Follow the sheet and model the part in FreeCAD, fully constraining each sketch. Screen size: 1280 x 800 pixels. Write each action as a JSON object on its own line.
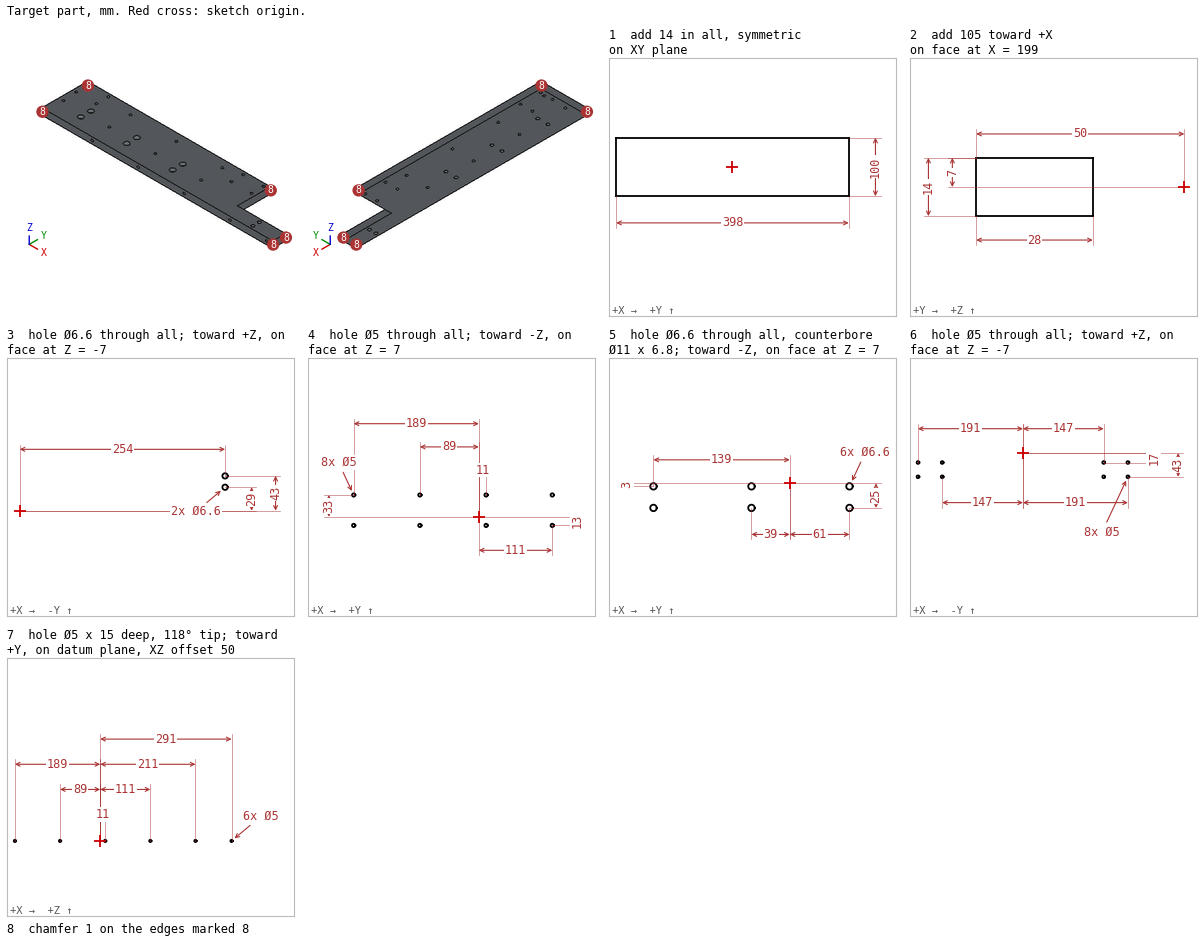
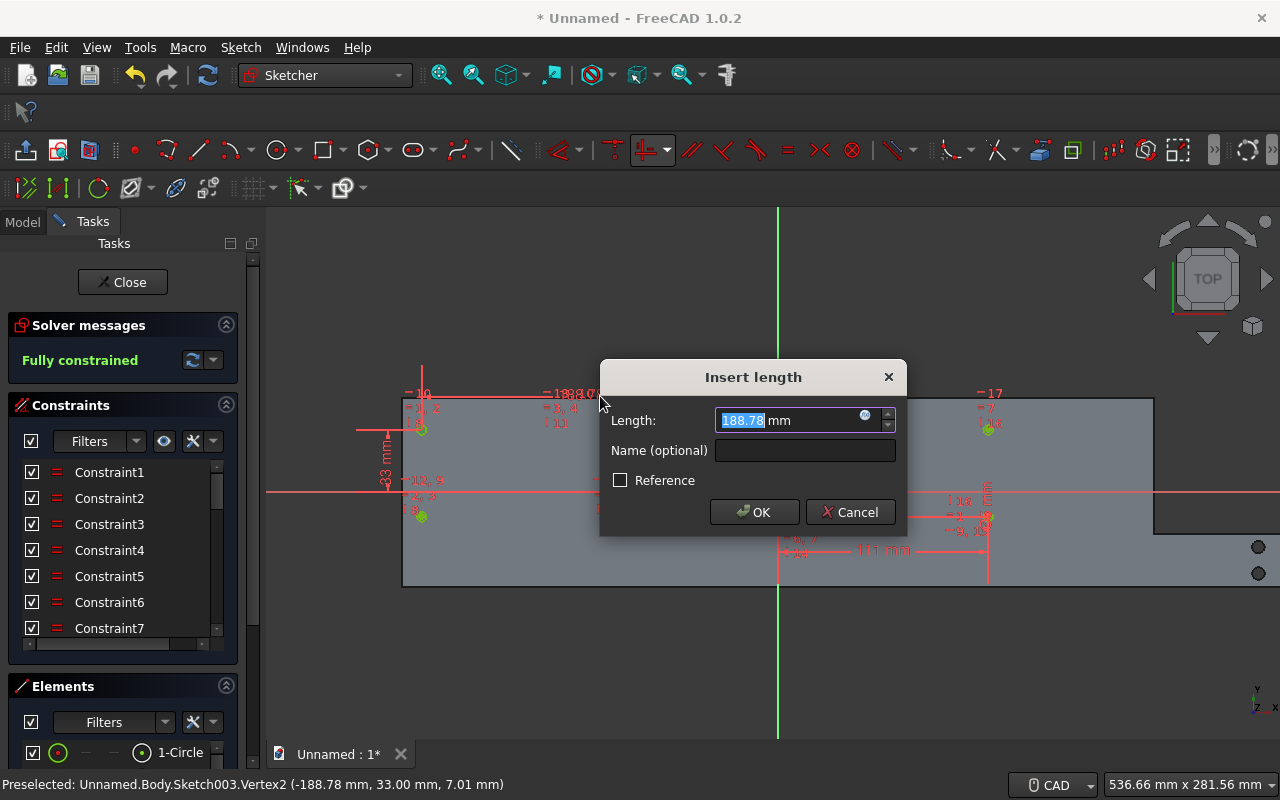
{"action": "type", "text": "189"}
{"action": "key", "text": "Return"}
{"action": "key", "text": "Escape"}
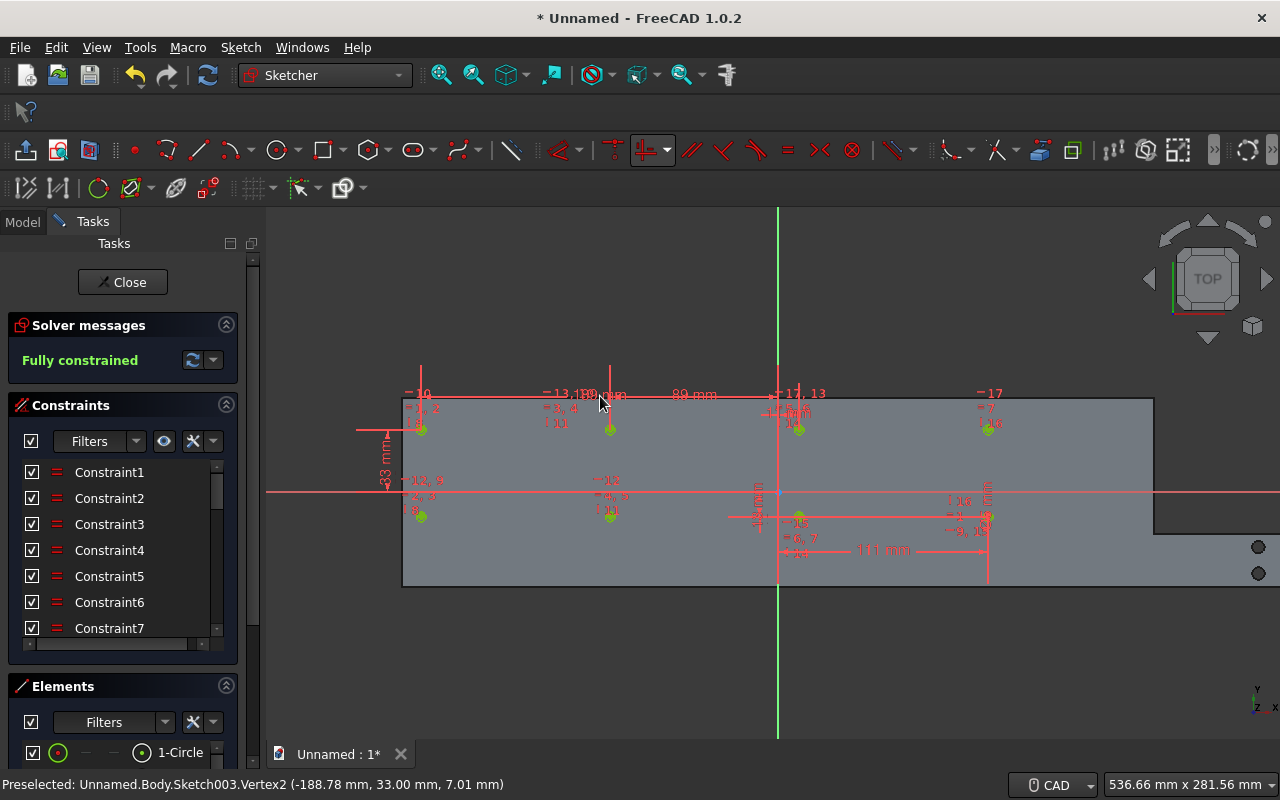
{"action": "left_click", "coordinate": [123, 282]}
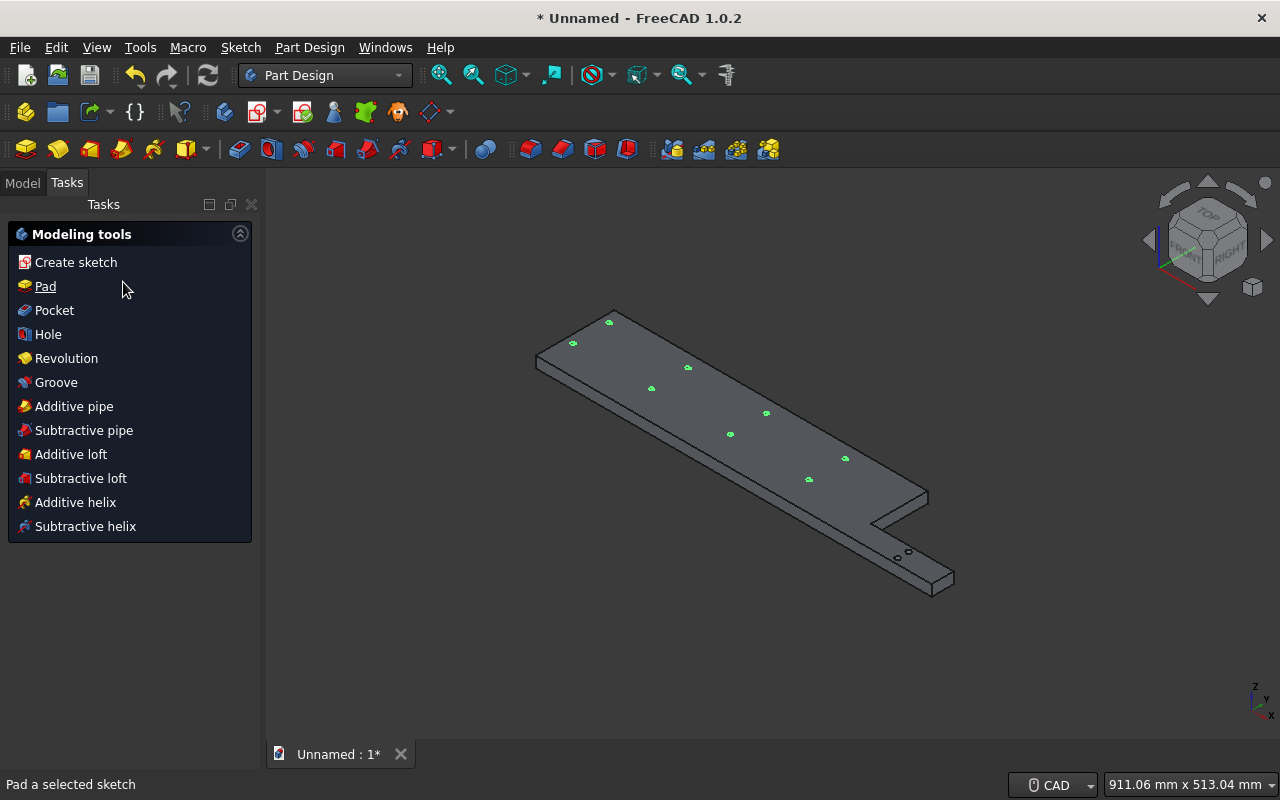
{"action": "left_click", "coordinate": [272, 150]}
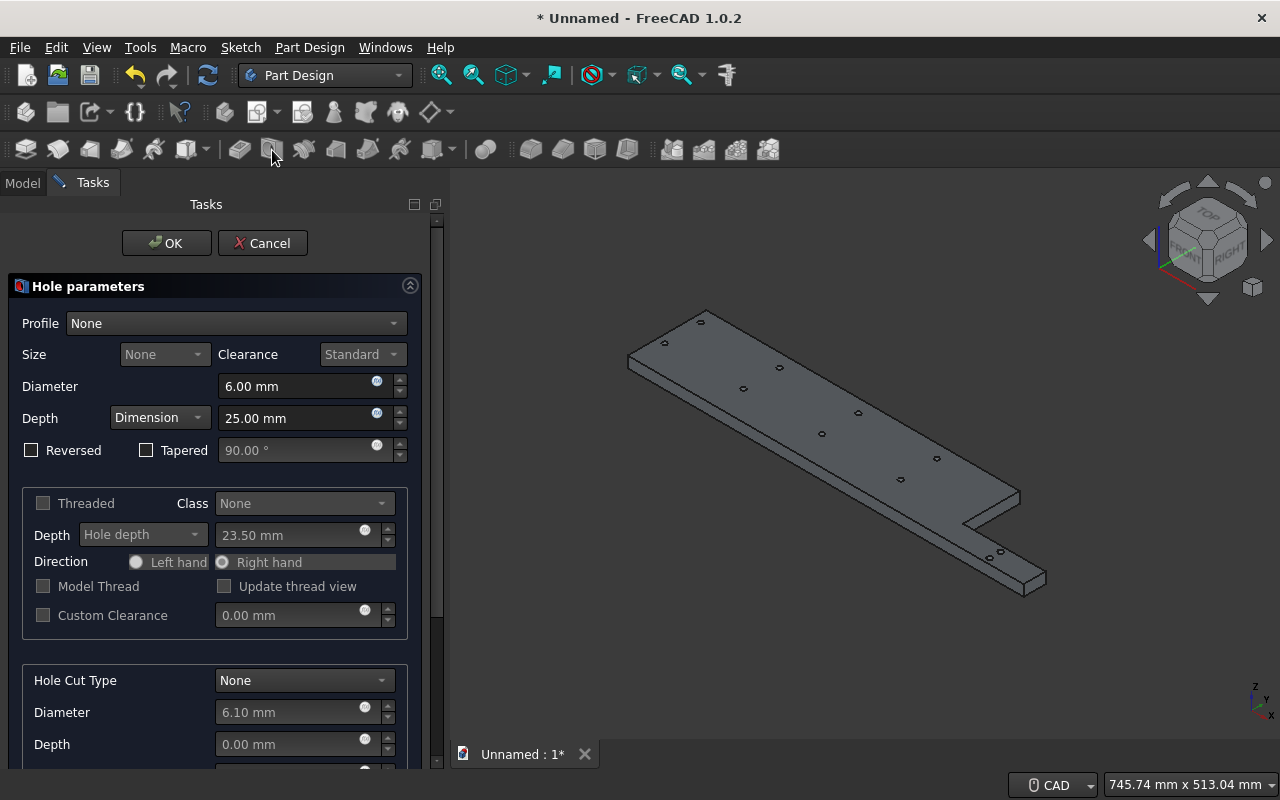
{"action": "triple_click", "coordinate": [305, 386]}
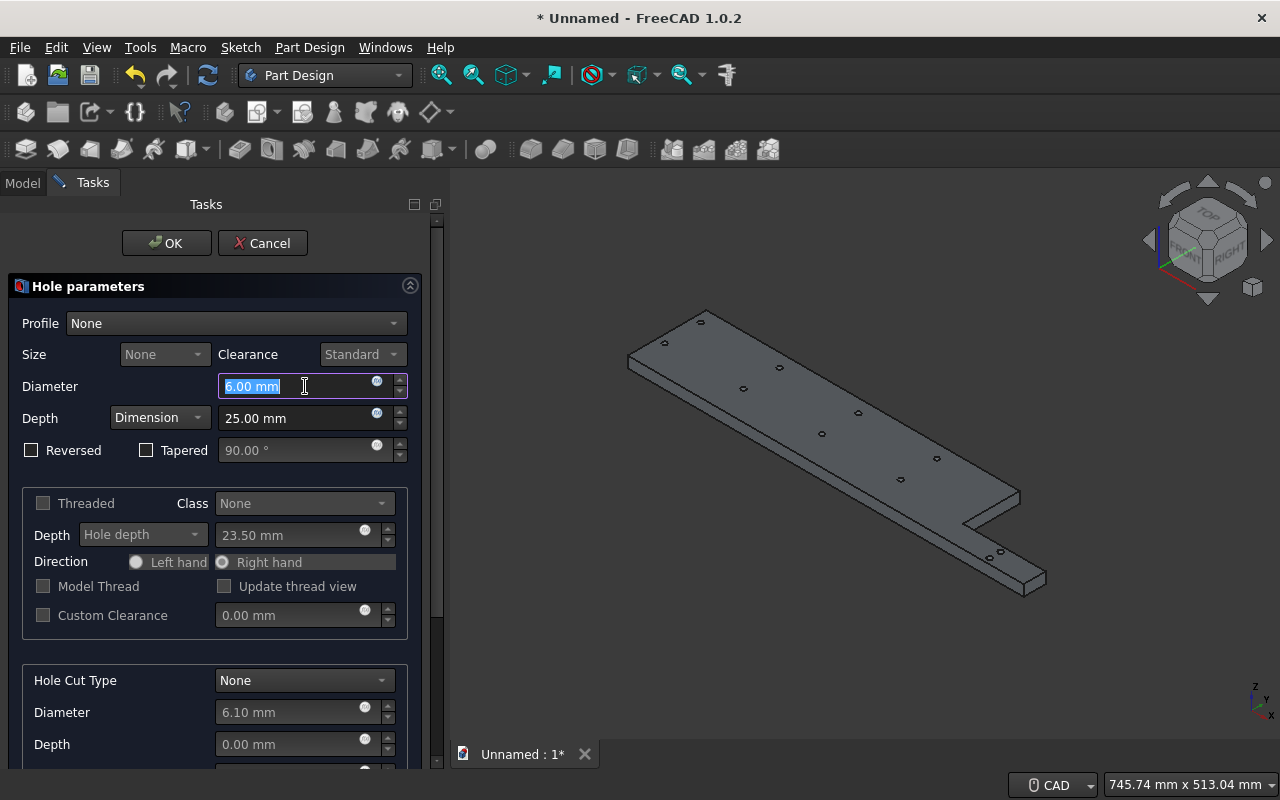
{"action": "type", "text": "5"}
{"action": "key", "text": "Tab"}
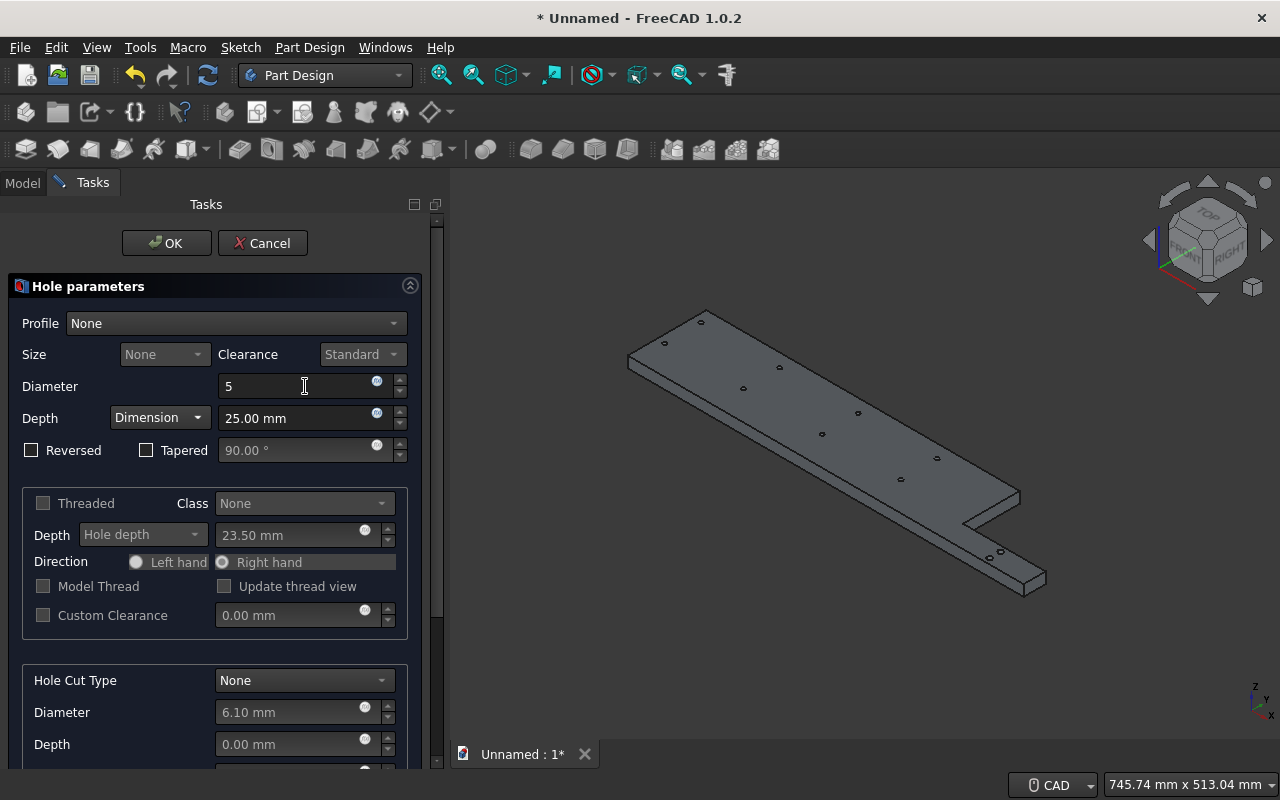
{"action": "left_click", "coordinate": [161, 418]}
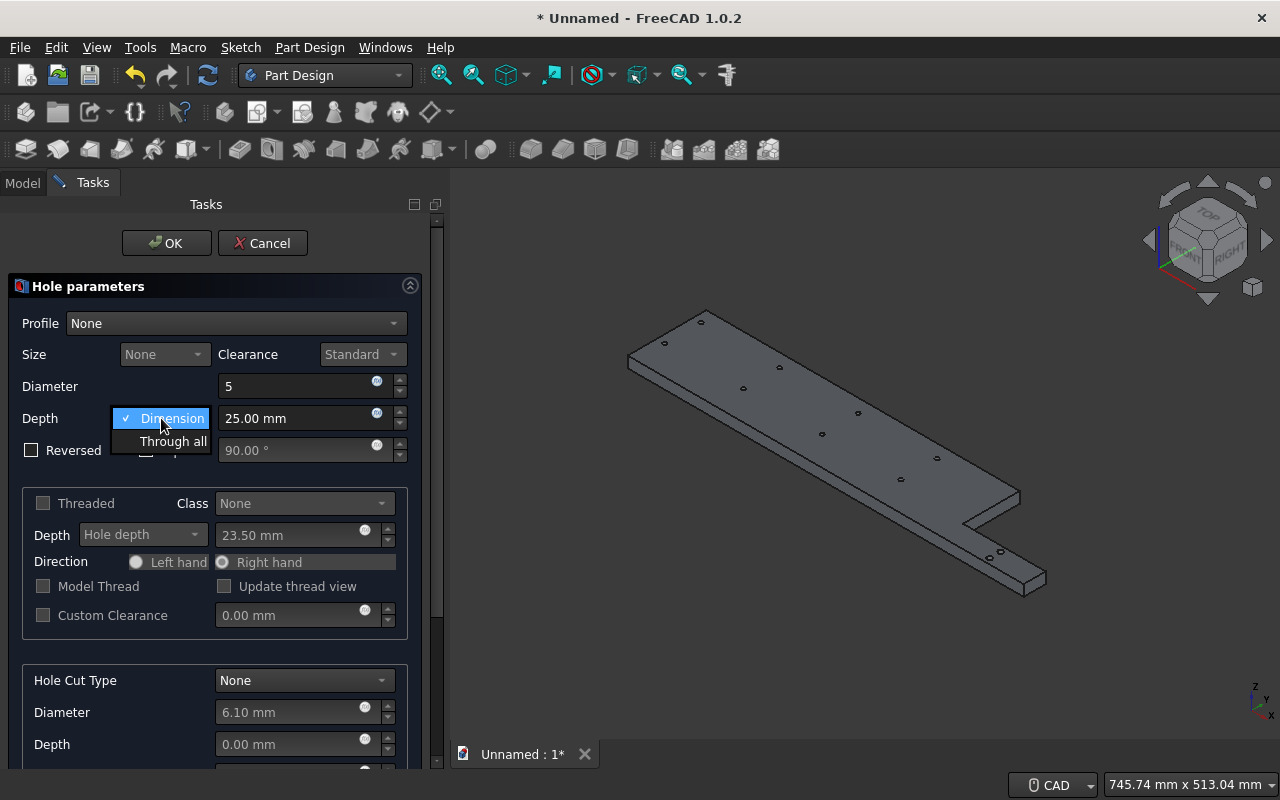
{"action": "left_click", "coordinate": [160, 442]}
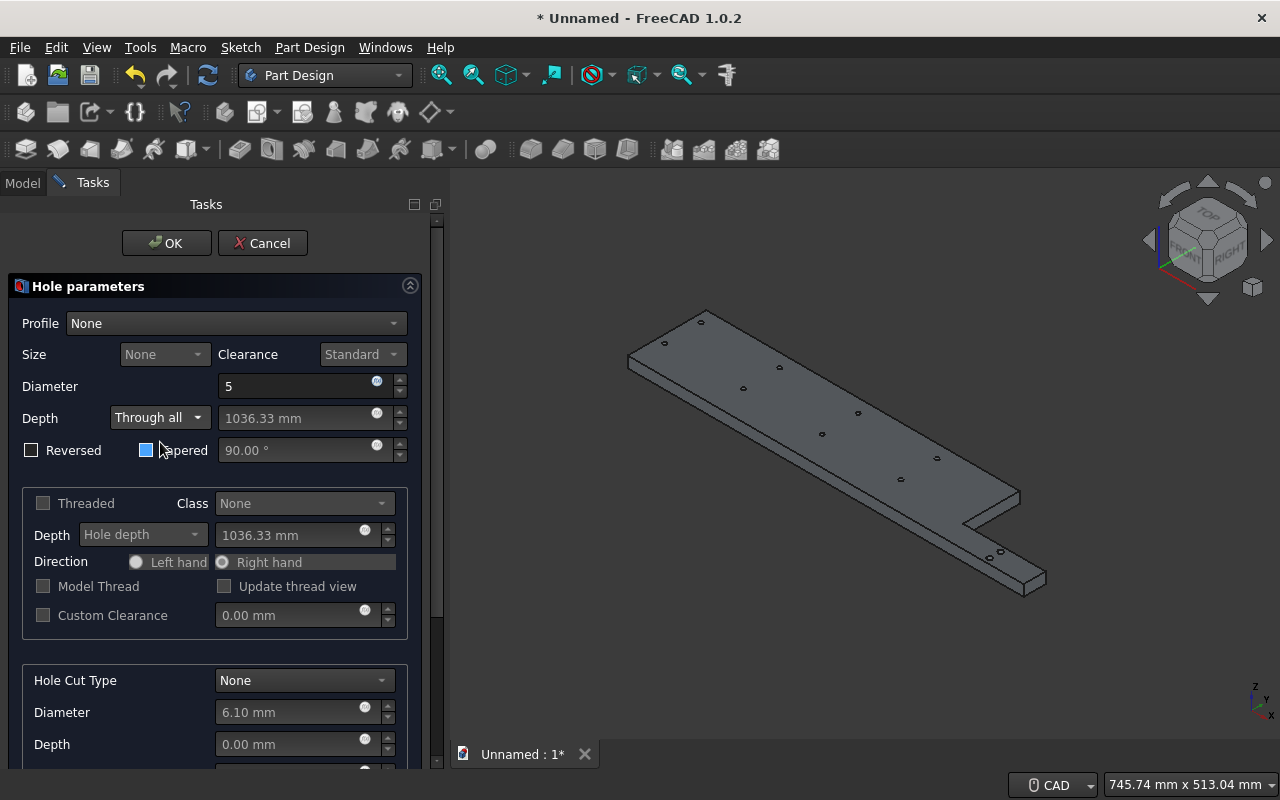
{"action": "left_click", "coordinate": [167, 243]}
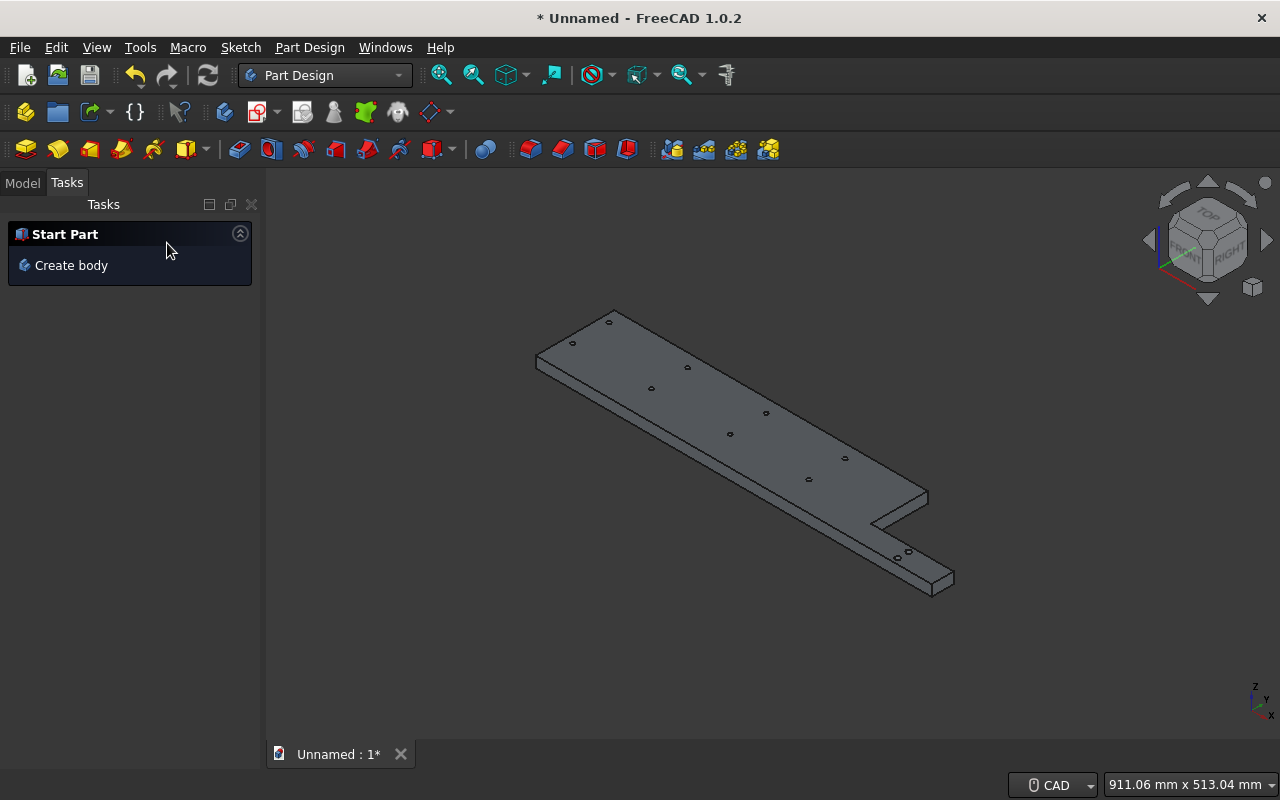
{"action": "left_click", "coordinate": [773, 446]}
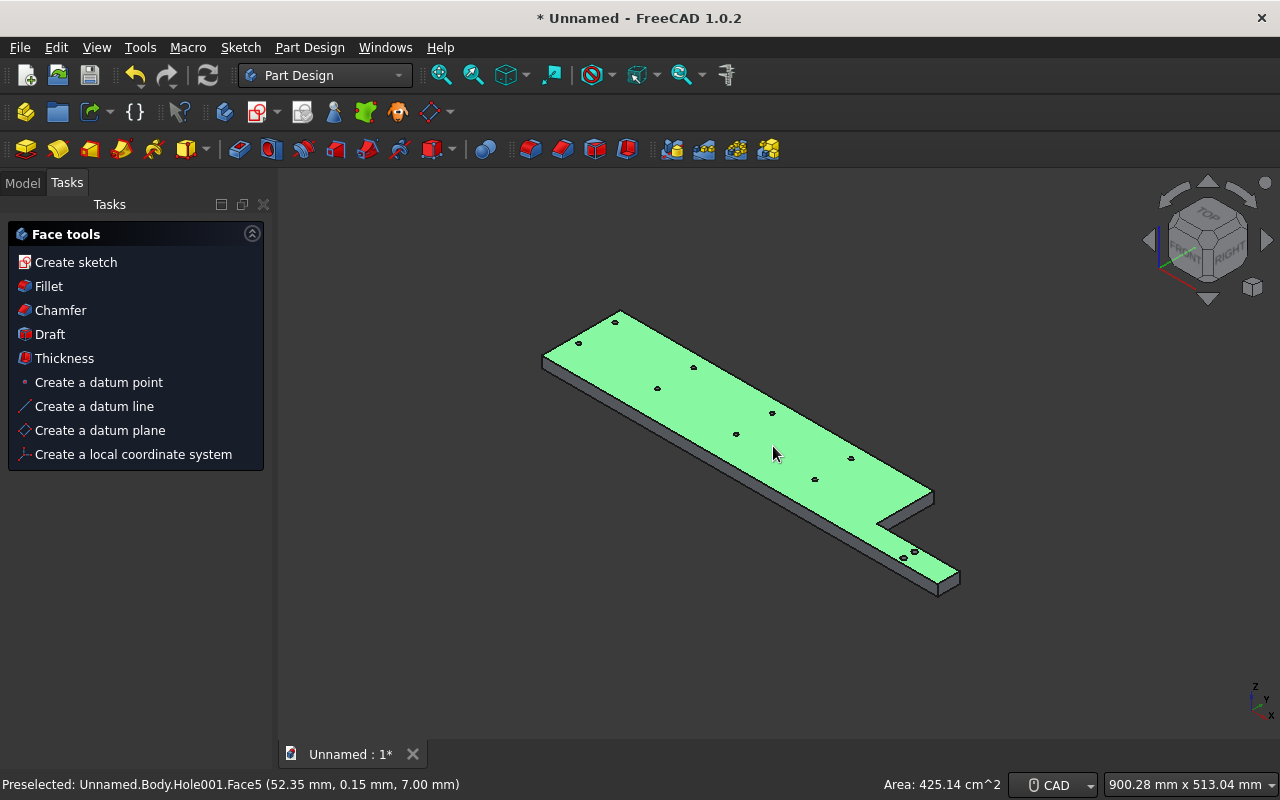
{"action": "left_click", "coordinate": [258, 112]}